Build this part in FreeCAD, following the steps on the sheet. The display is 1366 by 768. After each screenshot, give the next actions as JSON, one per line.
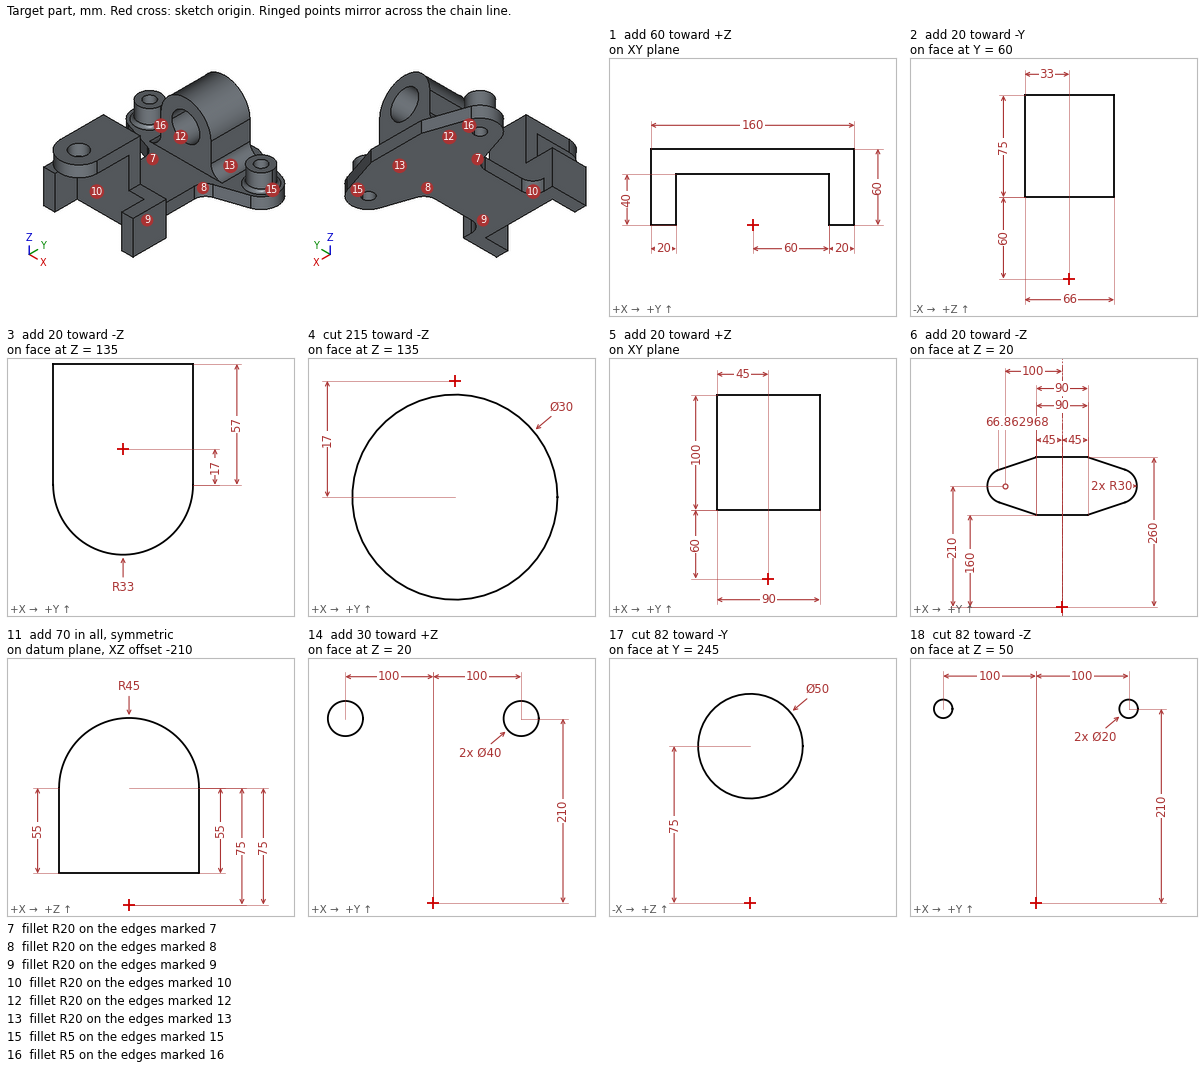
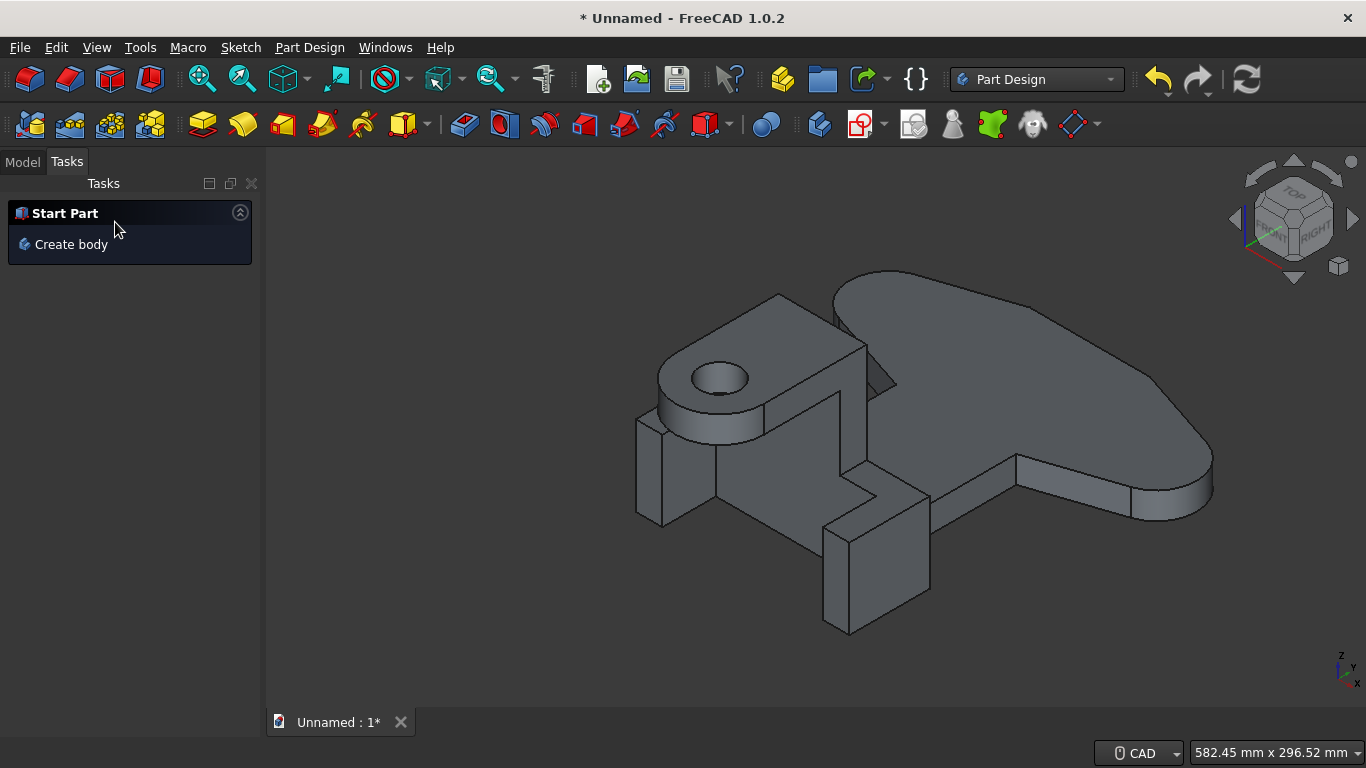
{"action": "key", "text": "2"}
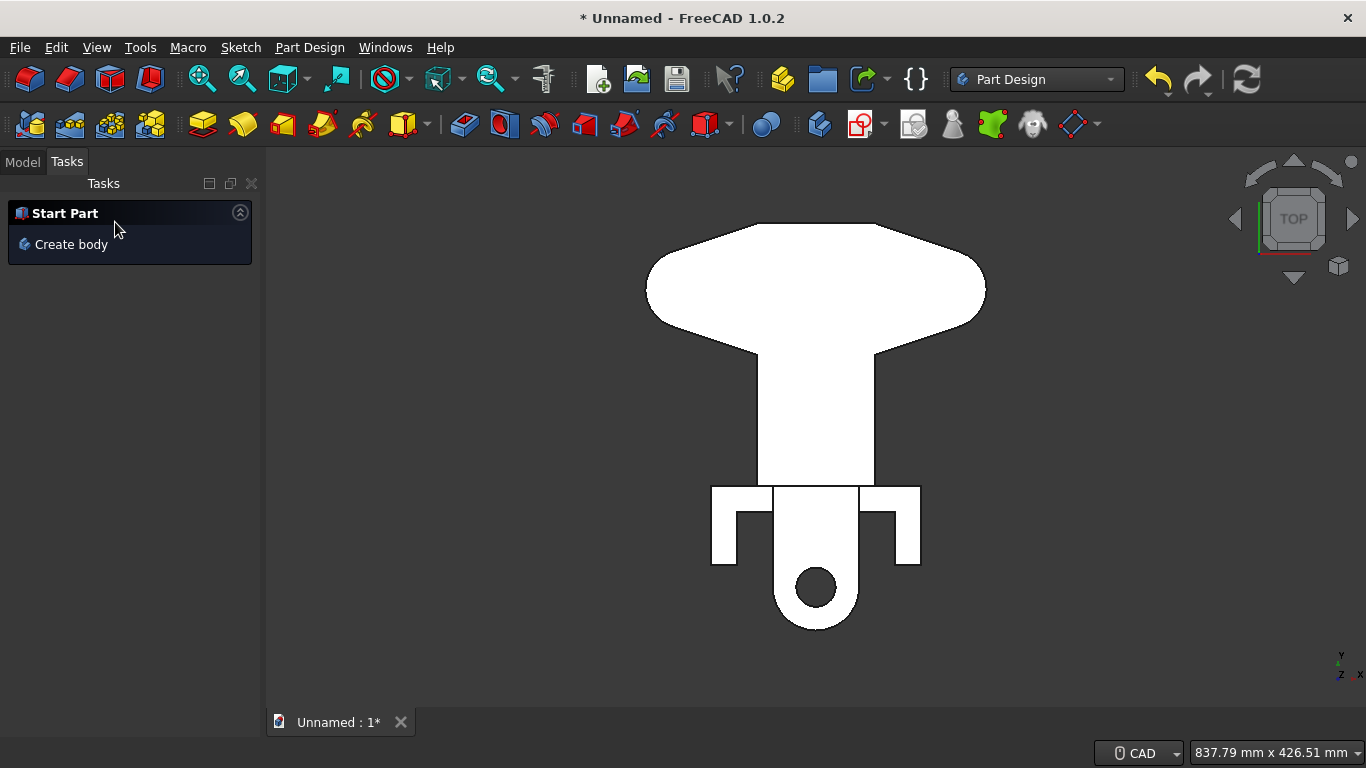
{"action": "key", "text": "0"}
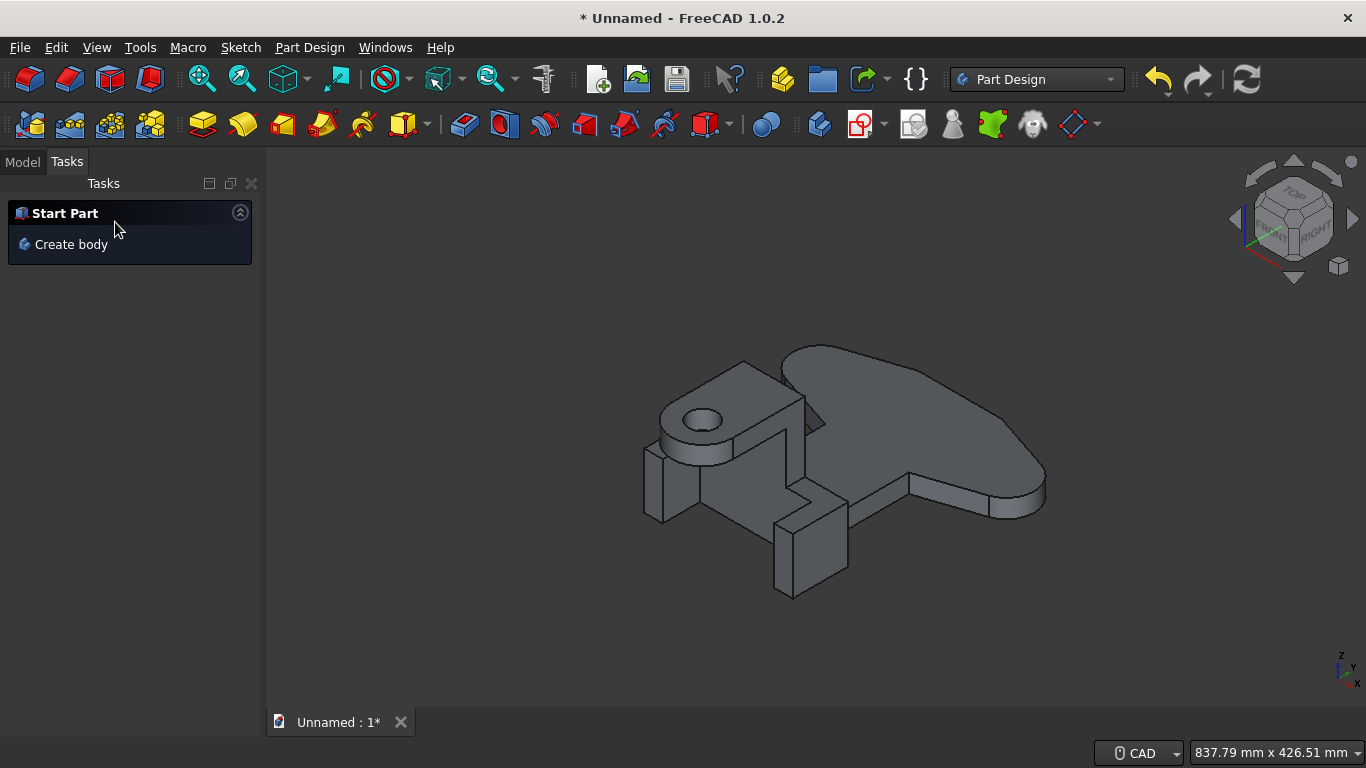
{"action": "key", "text": "1"}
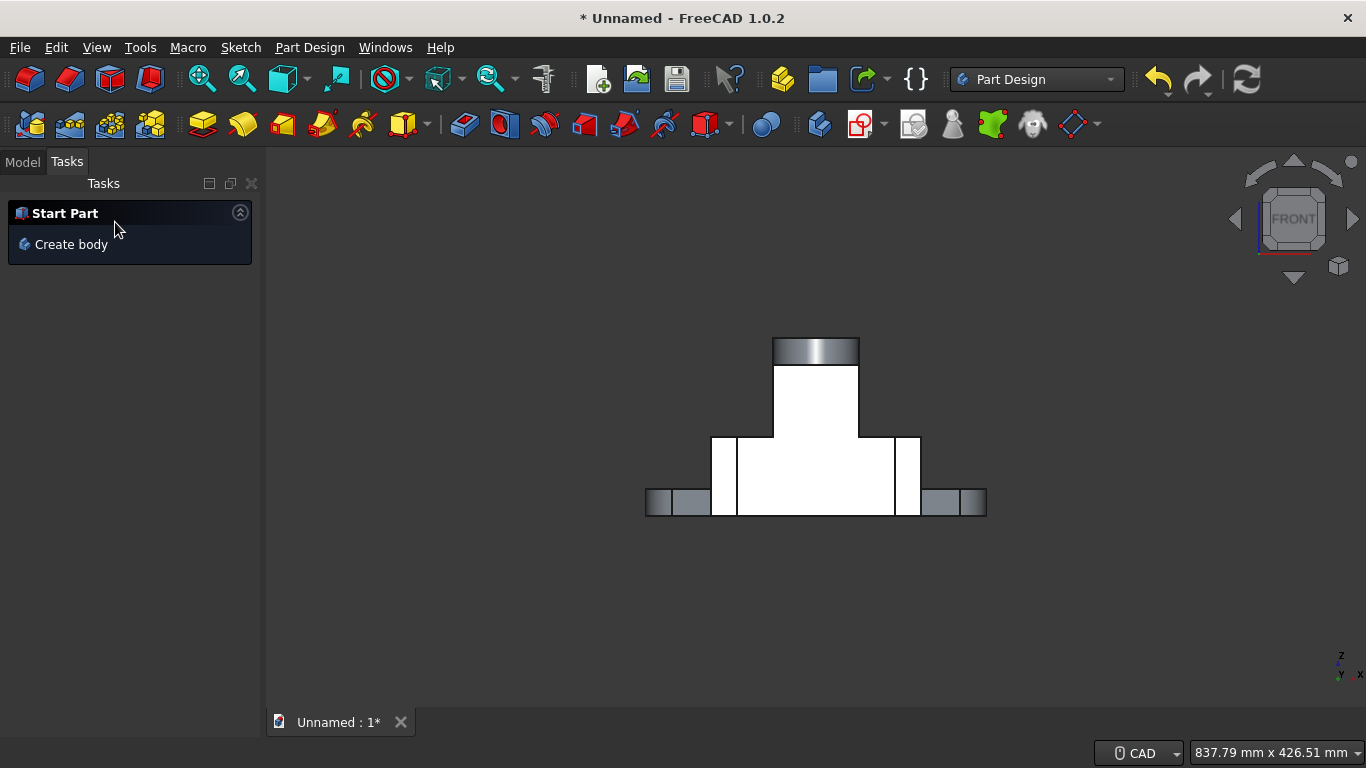
{"action": "key", "text": "v f"}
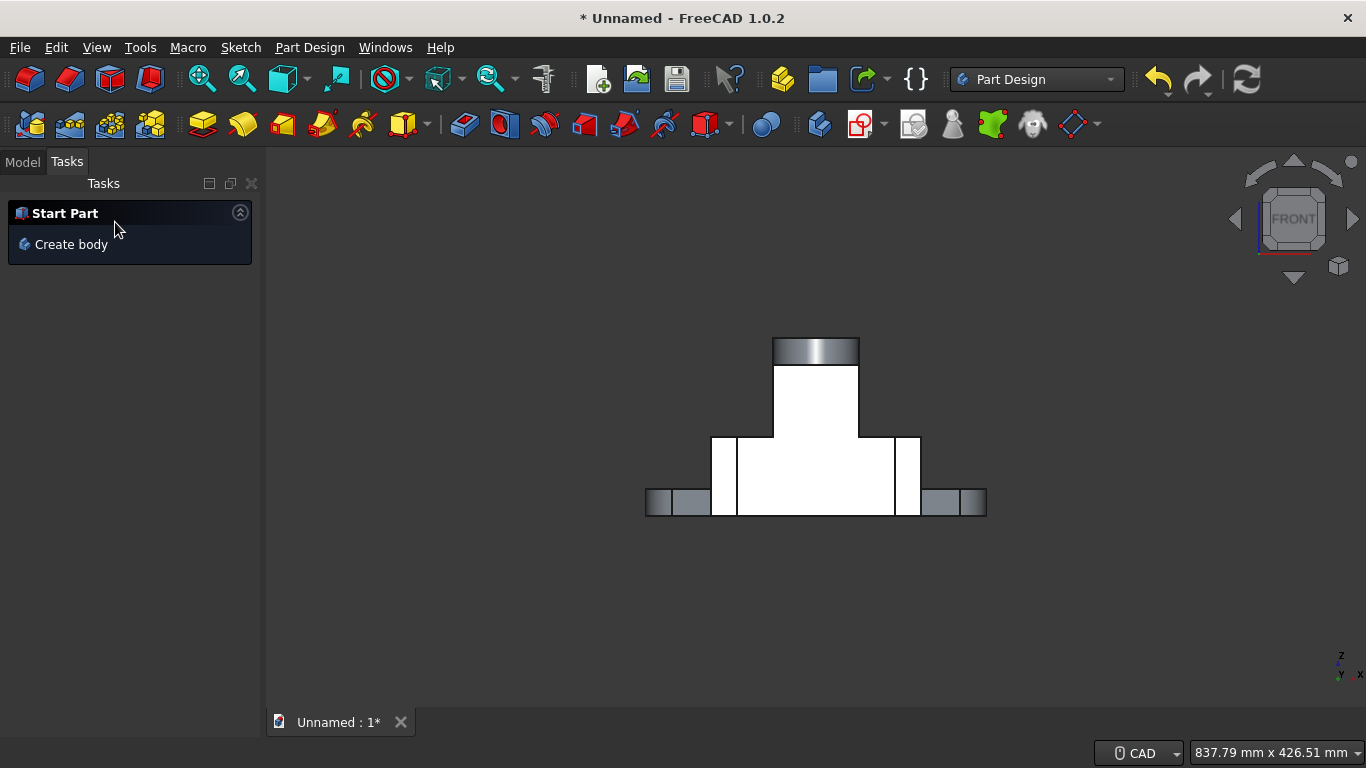
{"action": "key", "text": "3"}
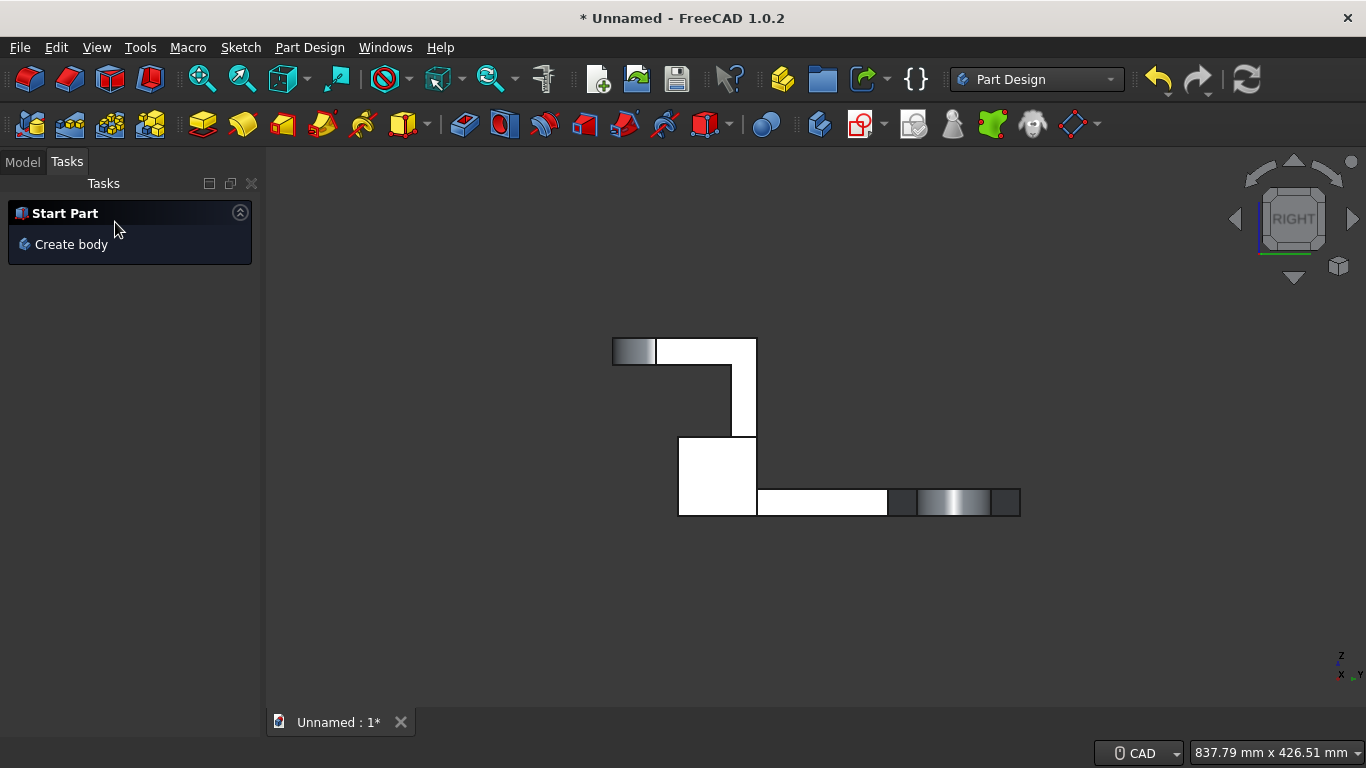
{"action": "key", "text": "v f"}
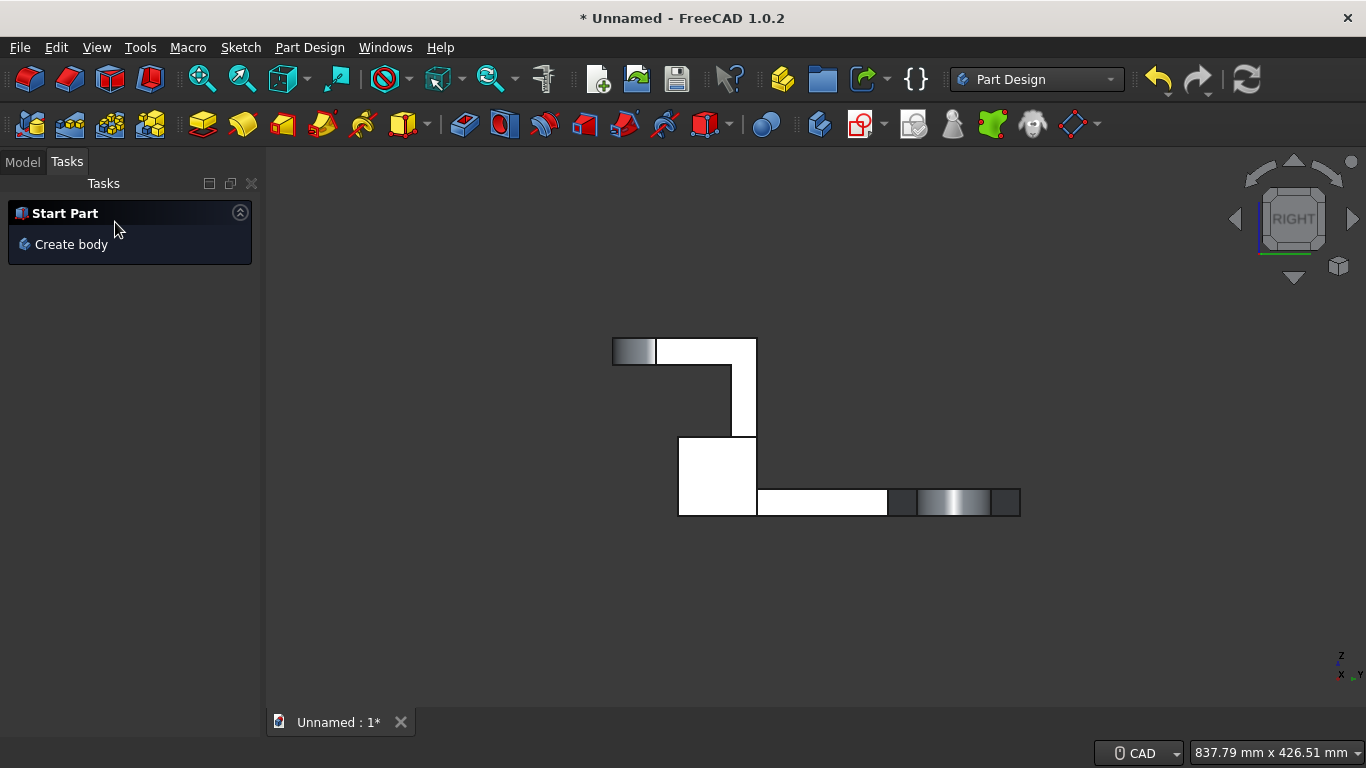
{"action": "key", "text": "5"}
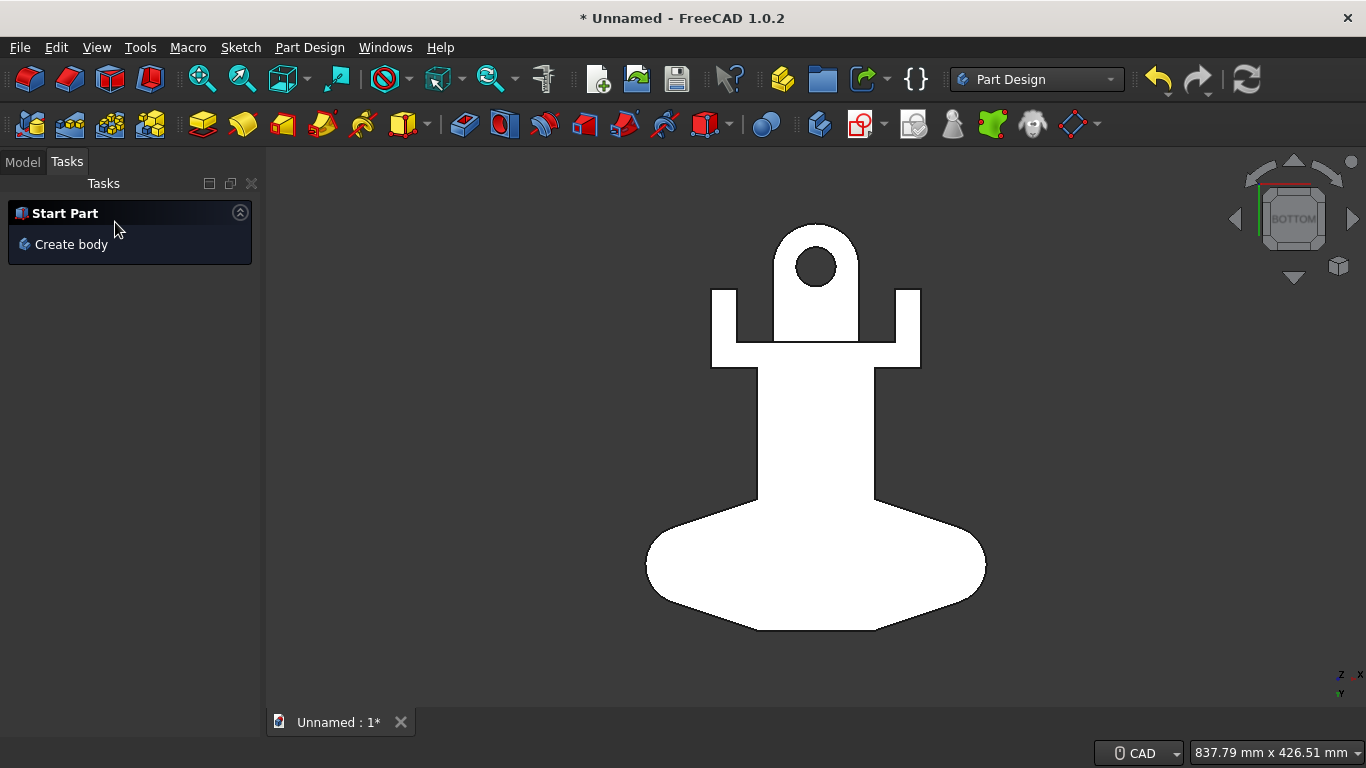
{"action": "key", "text": "4"}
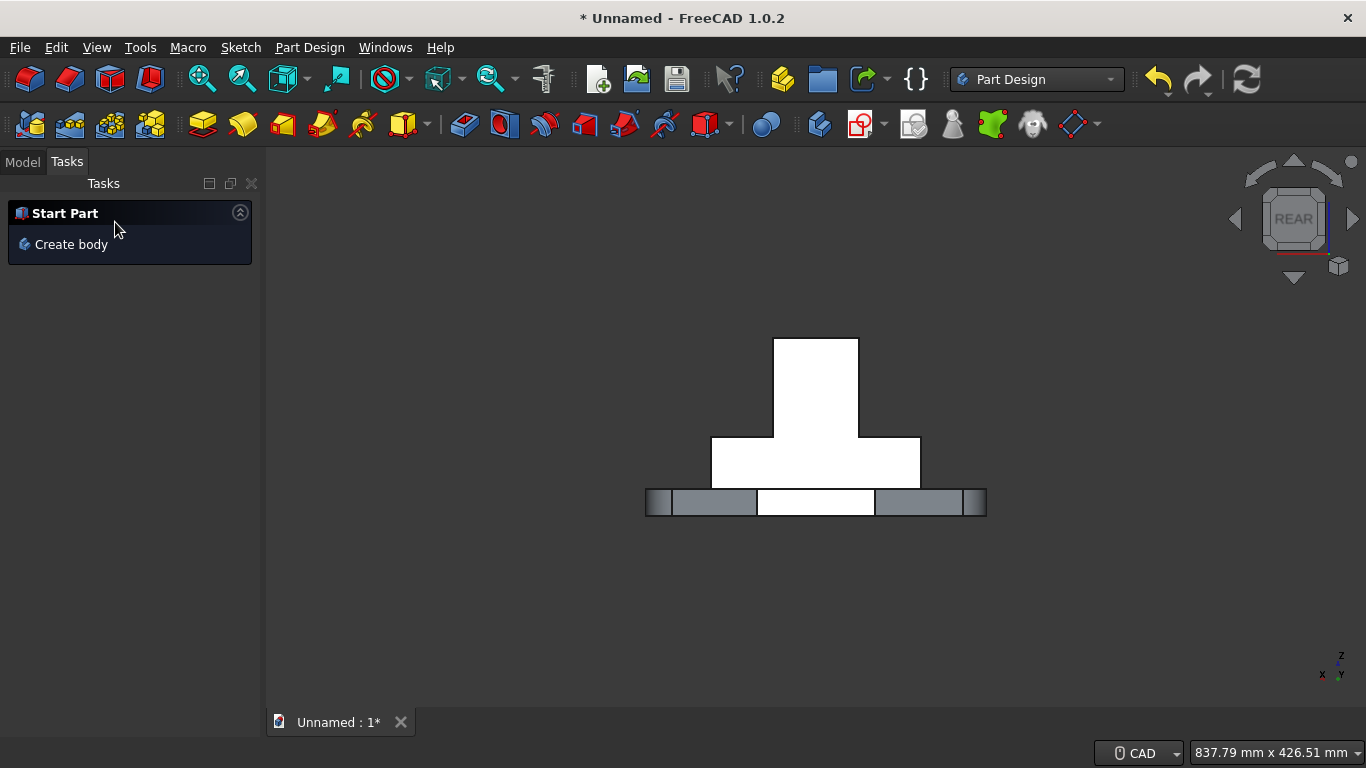
{"action": "key", "text": "v f"}